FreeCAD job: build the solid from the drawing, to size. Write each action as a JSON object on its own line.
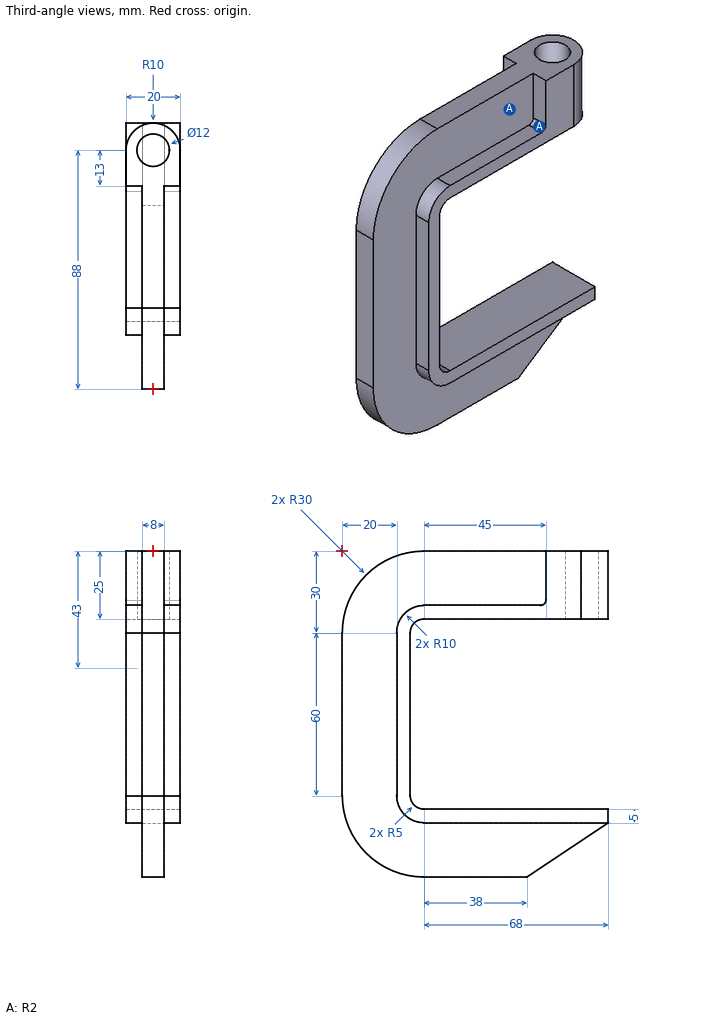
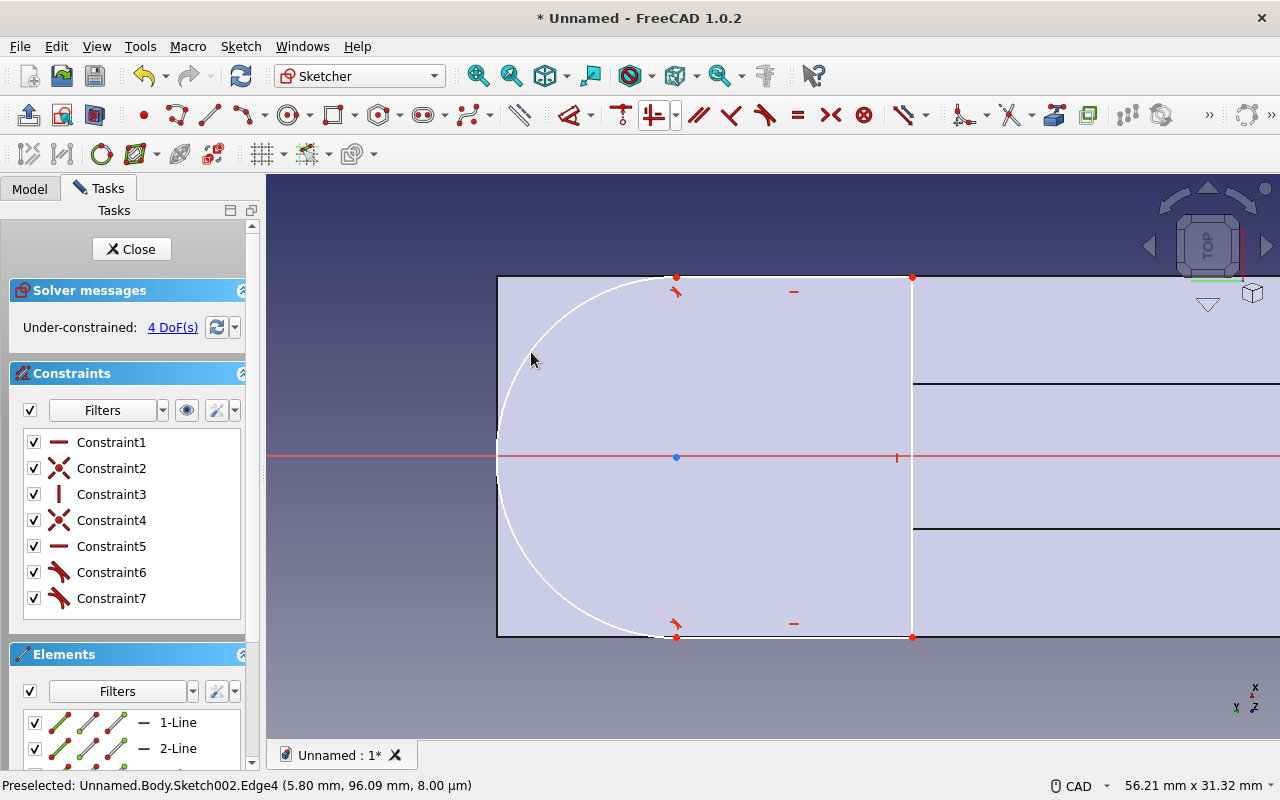
{"action": "left_click", "coordinate": [677, 458]}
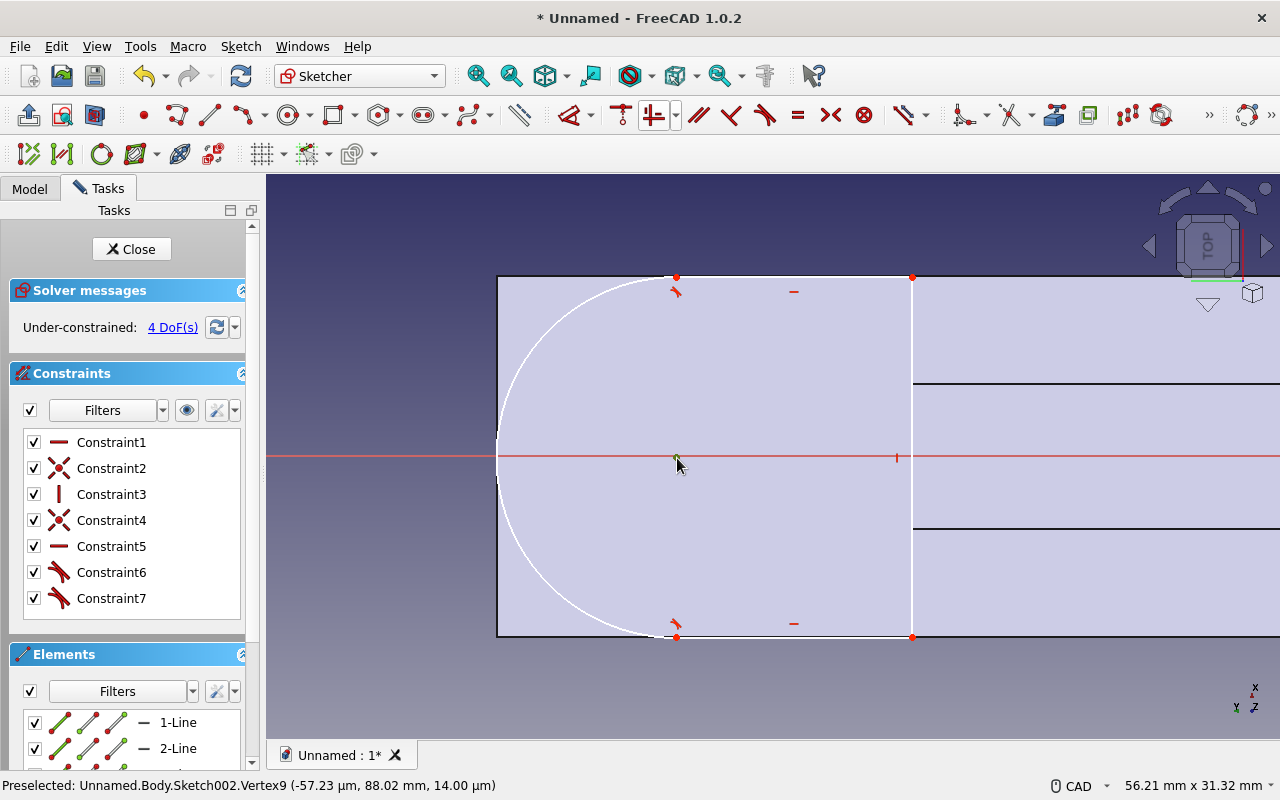
{"action": "left_click", "coordinate": [353, 456]}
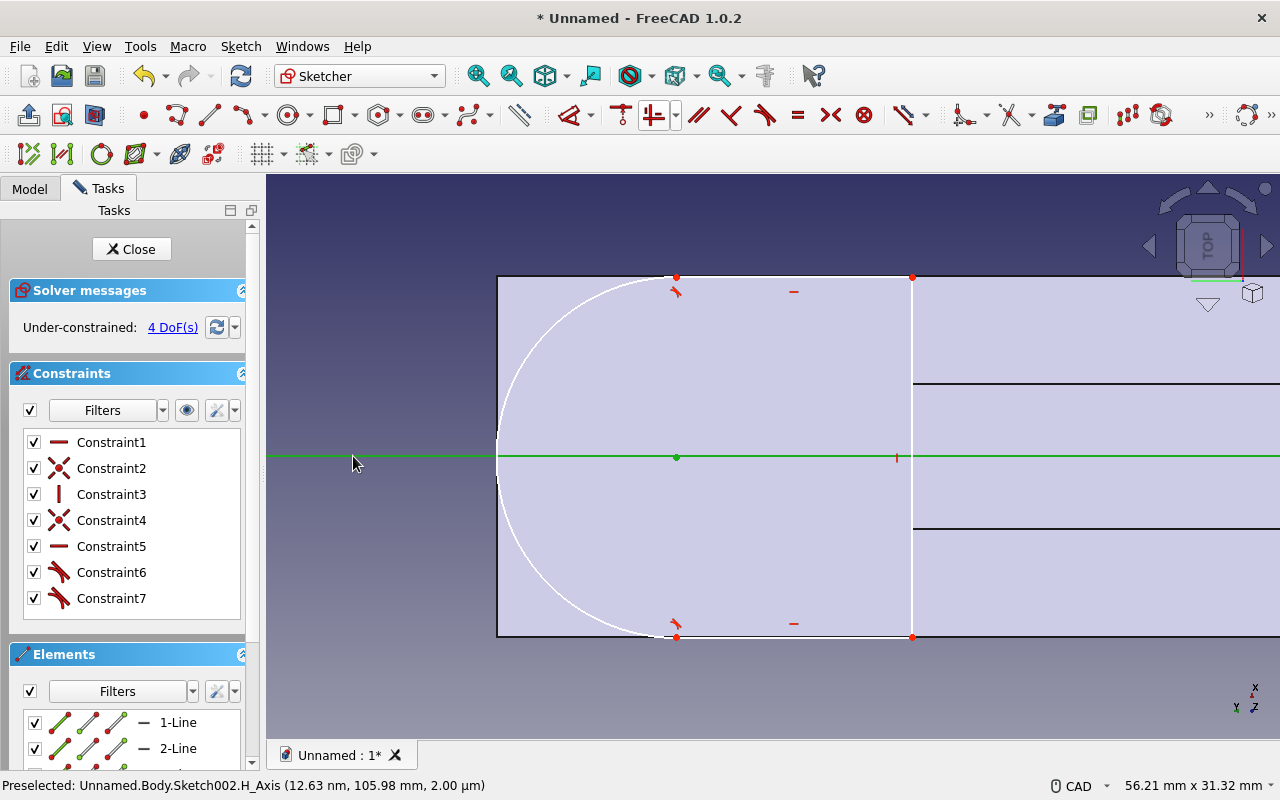
{"action": "key", "text": "c"}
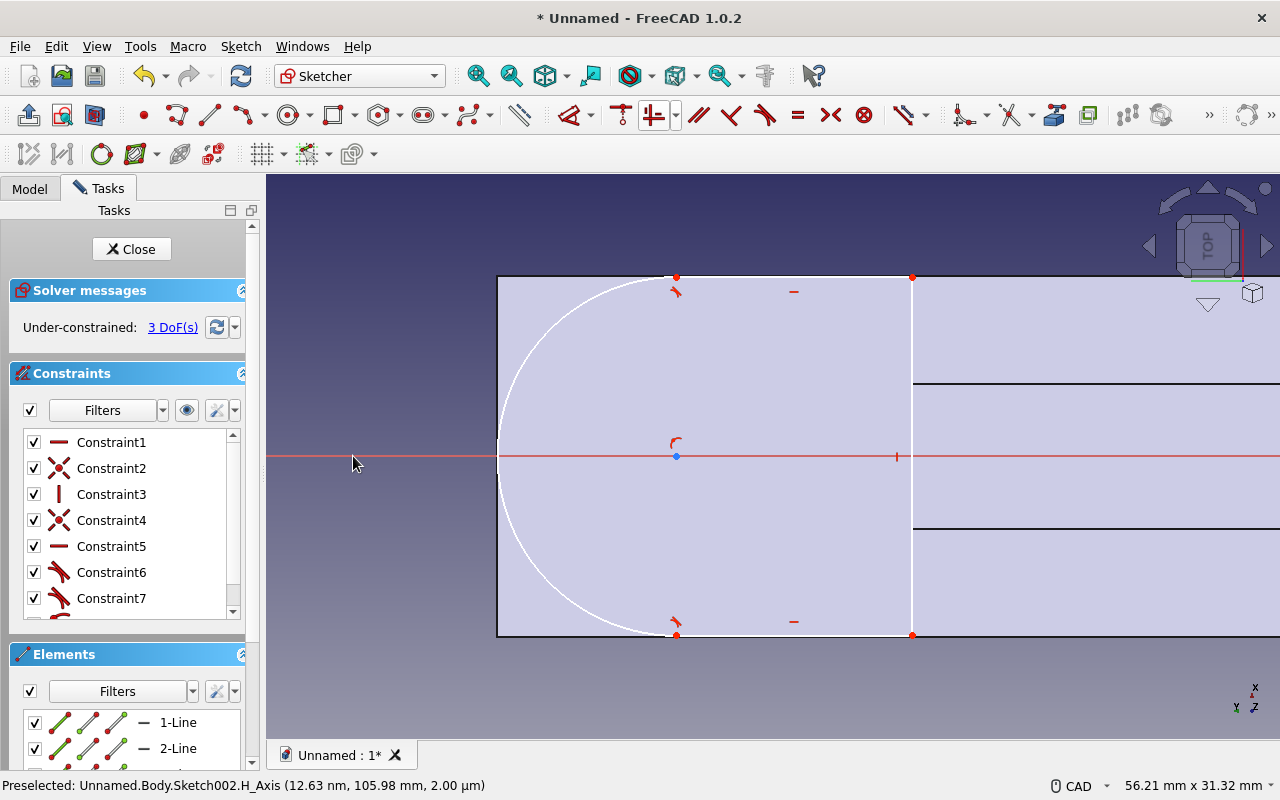
{"action": "left_click", "coordinate": [568, 116]}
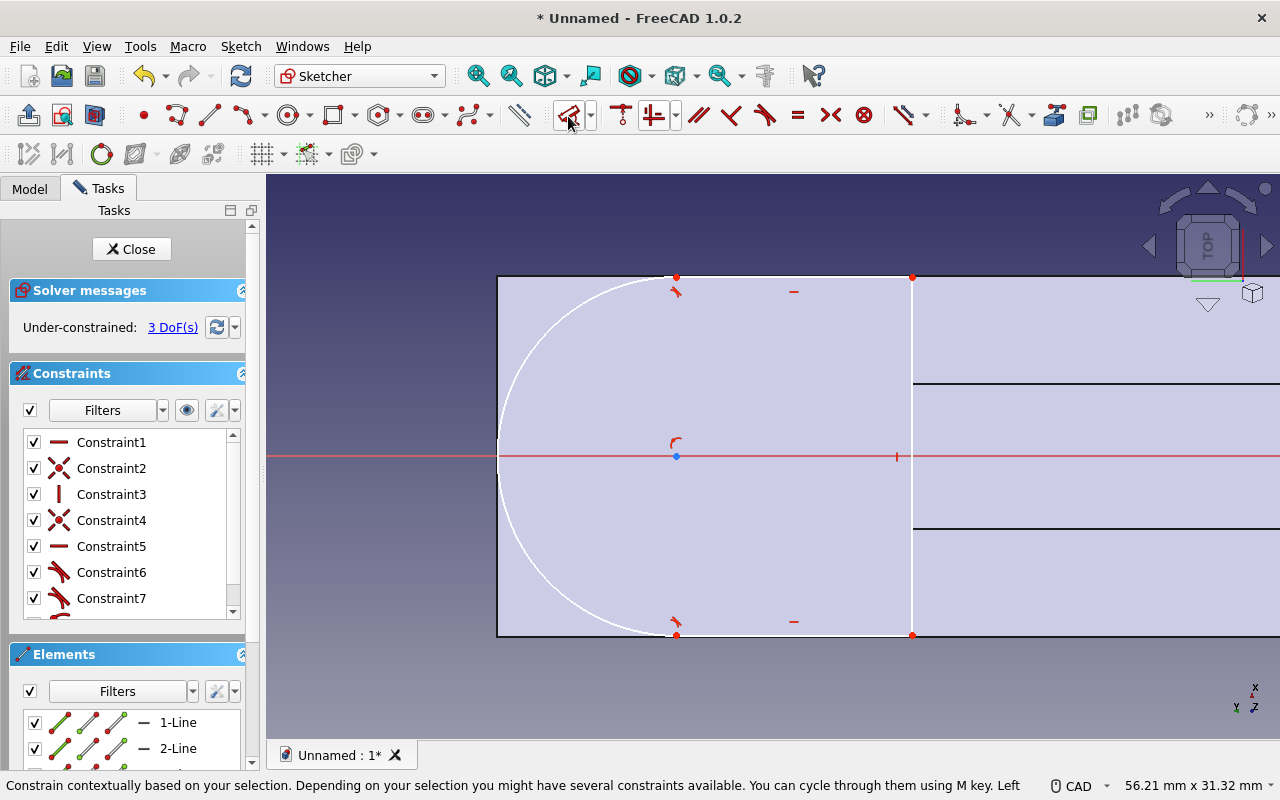
{"action": "left_click", "coordinate": [532, 351]}
{"action": "left_click", "coordinate": [506, 332]}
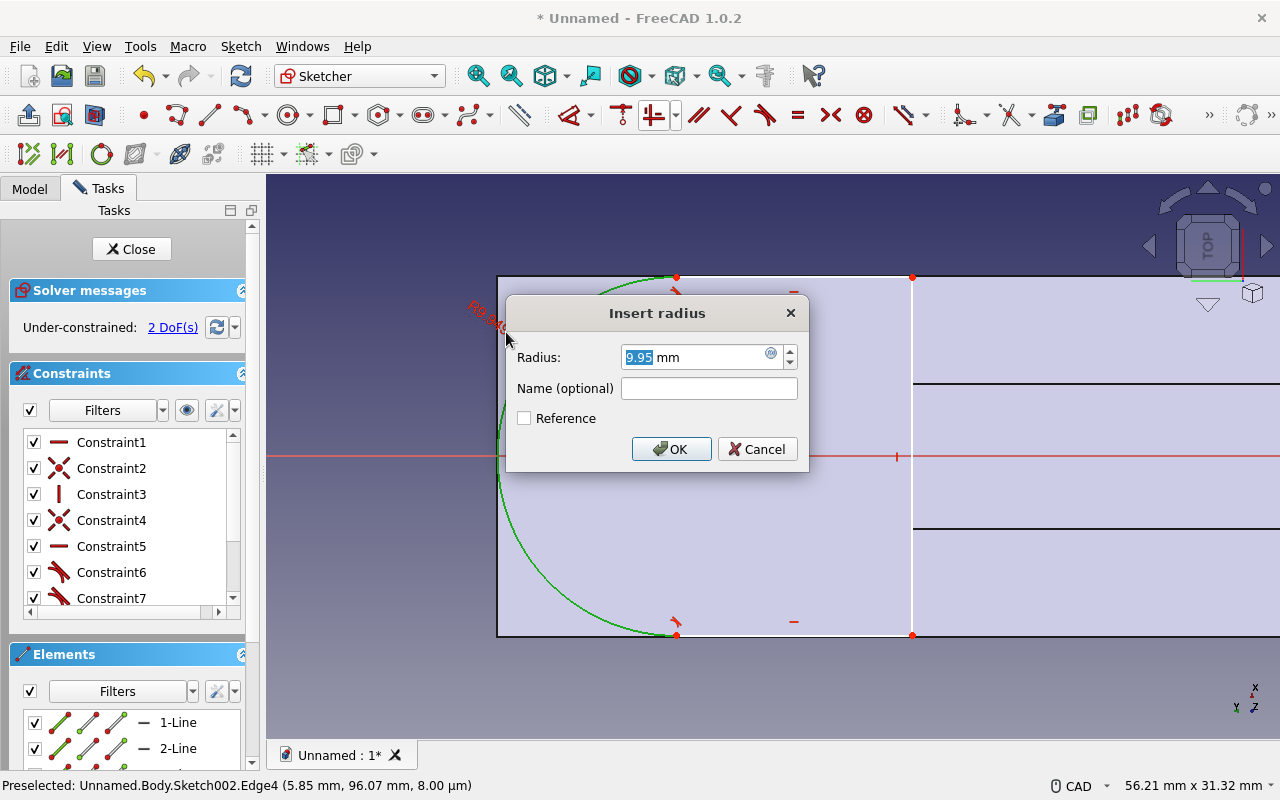
{"action": "type", "text": "10"}
{"action": "key", "text": "Return"}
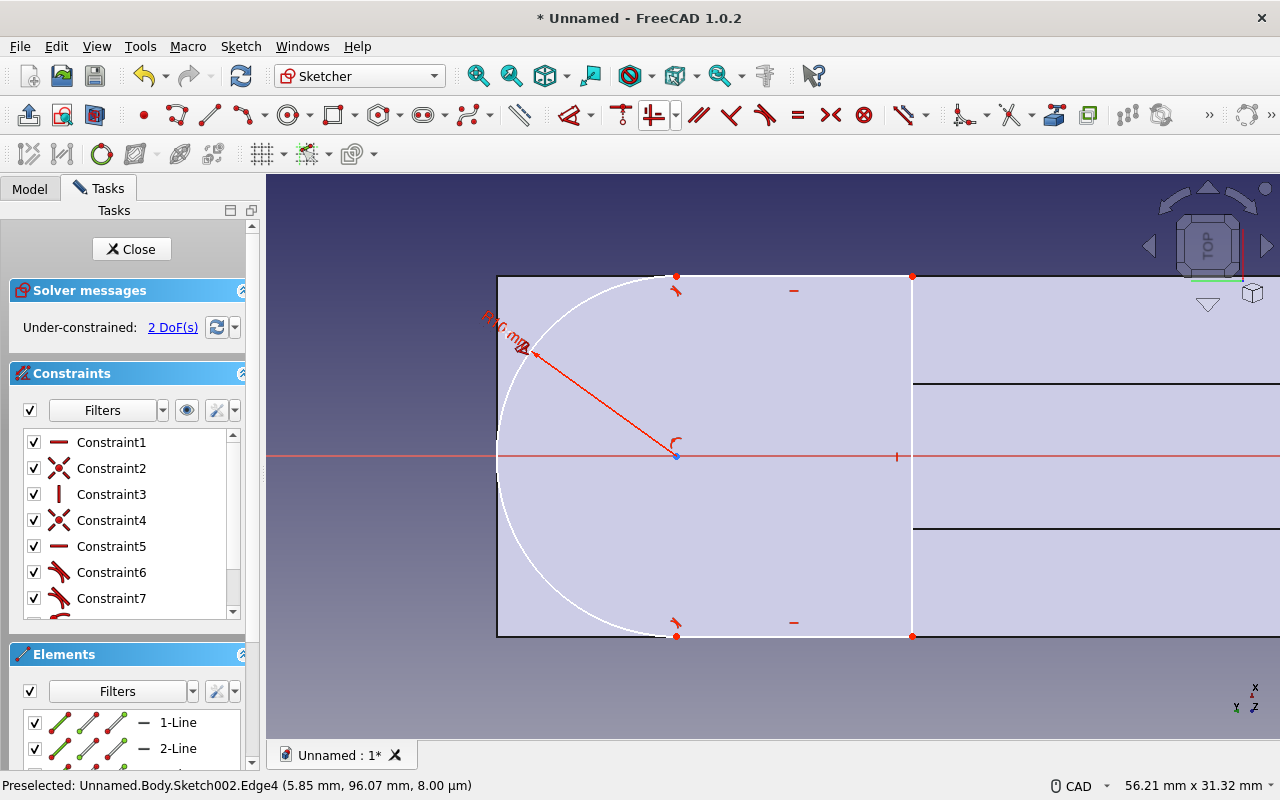
{"action": "left_click", "coordinate": [748, 637]}
{"action": "left_click", "coordinate": [795, 671]}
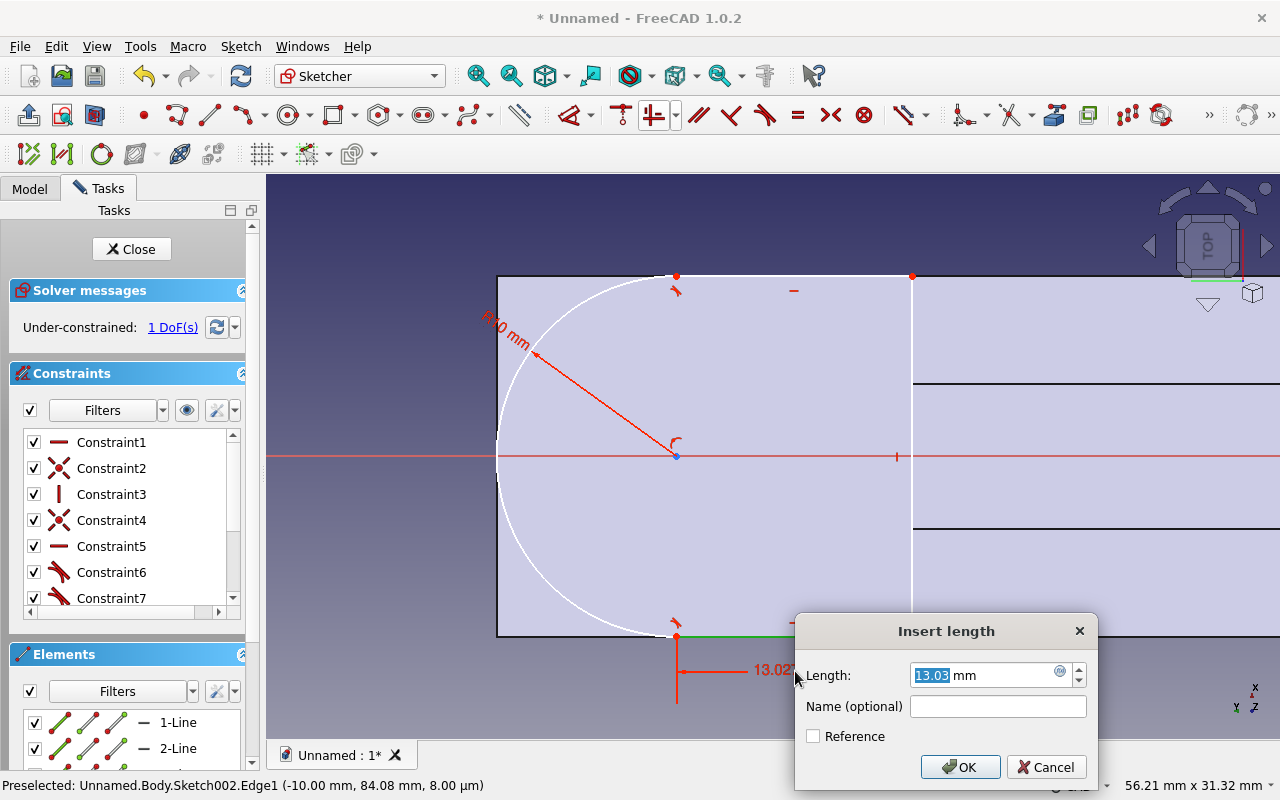
{"action": "type", "text": "13"}
{"action": "key", "text": "Return"}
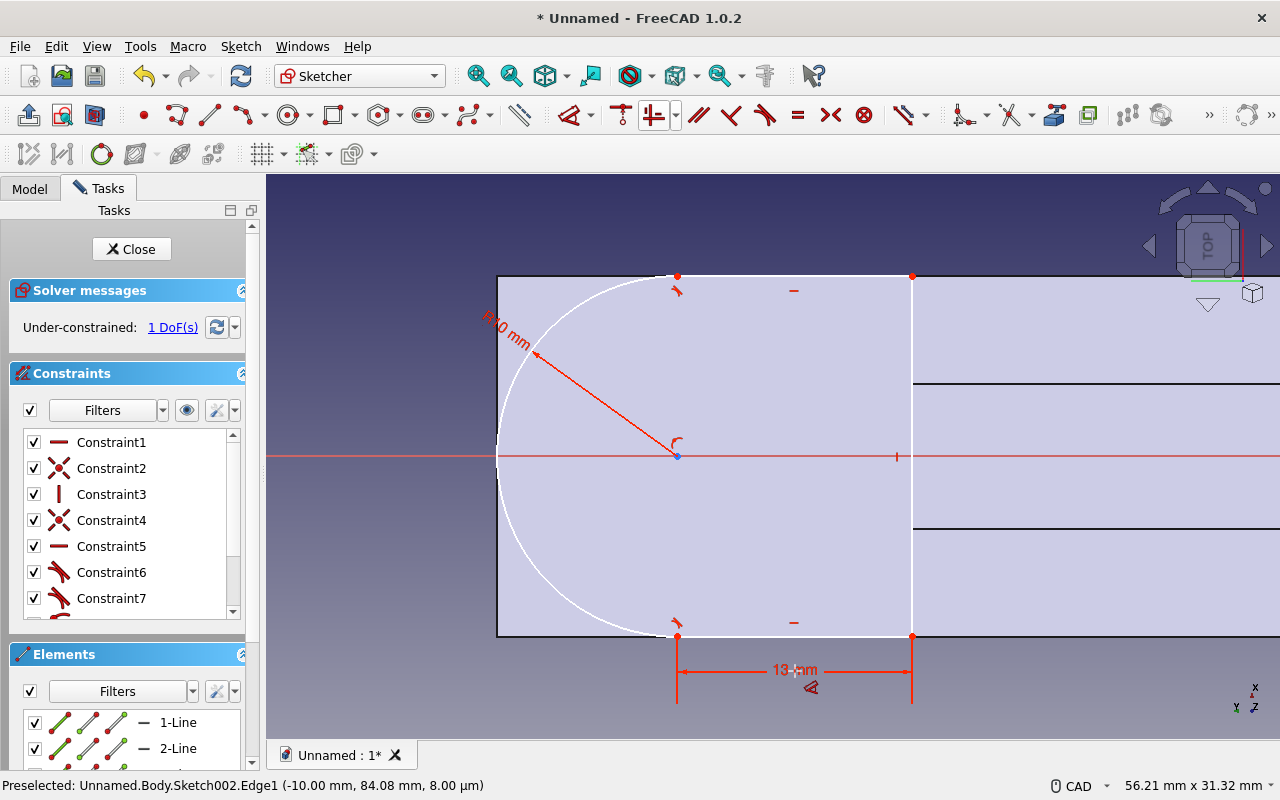
{"action": "left_click", "coordinate": [677, 637]}
{"action": "left_click", "coordinate": [896, 671]}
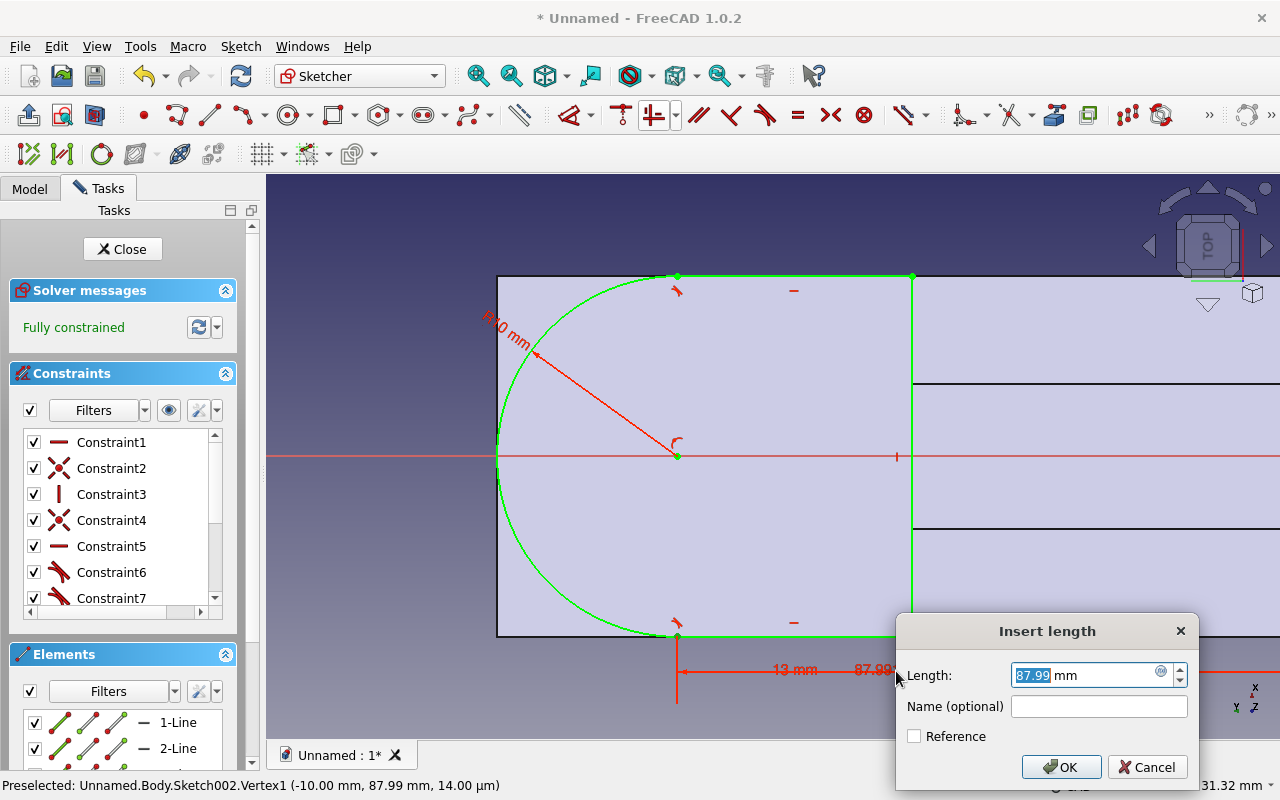
{"action": "type", "text": "88"}
{"action": "key", "text": "Return"}
{"action": "key", "text": "Escape"}